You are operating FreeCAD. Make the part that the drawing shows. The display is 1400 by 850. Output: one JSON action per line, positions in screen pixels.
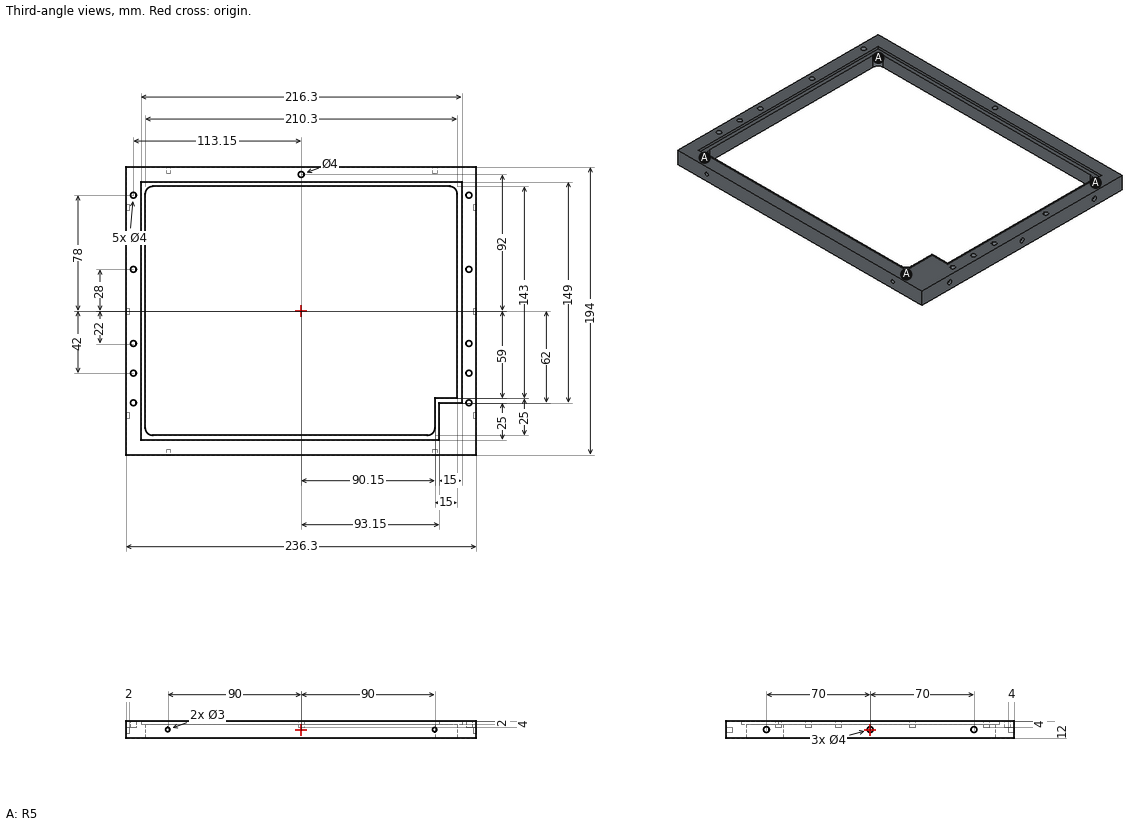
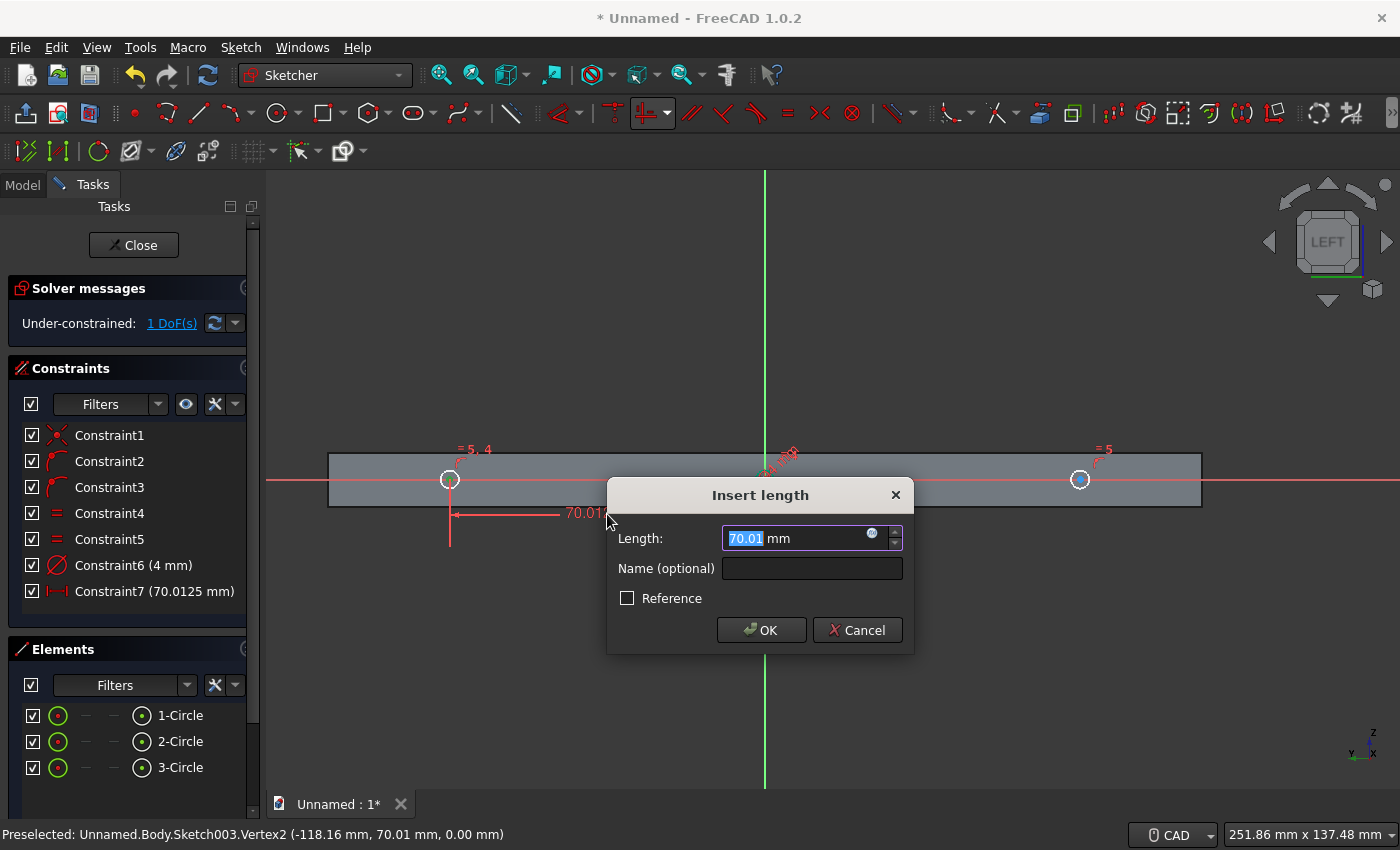
{"action": "type", "text": "70"}
{"action": "key", "text": "Return"}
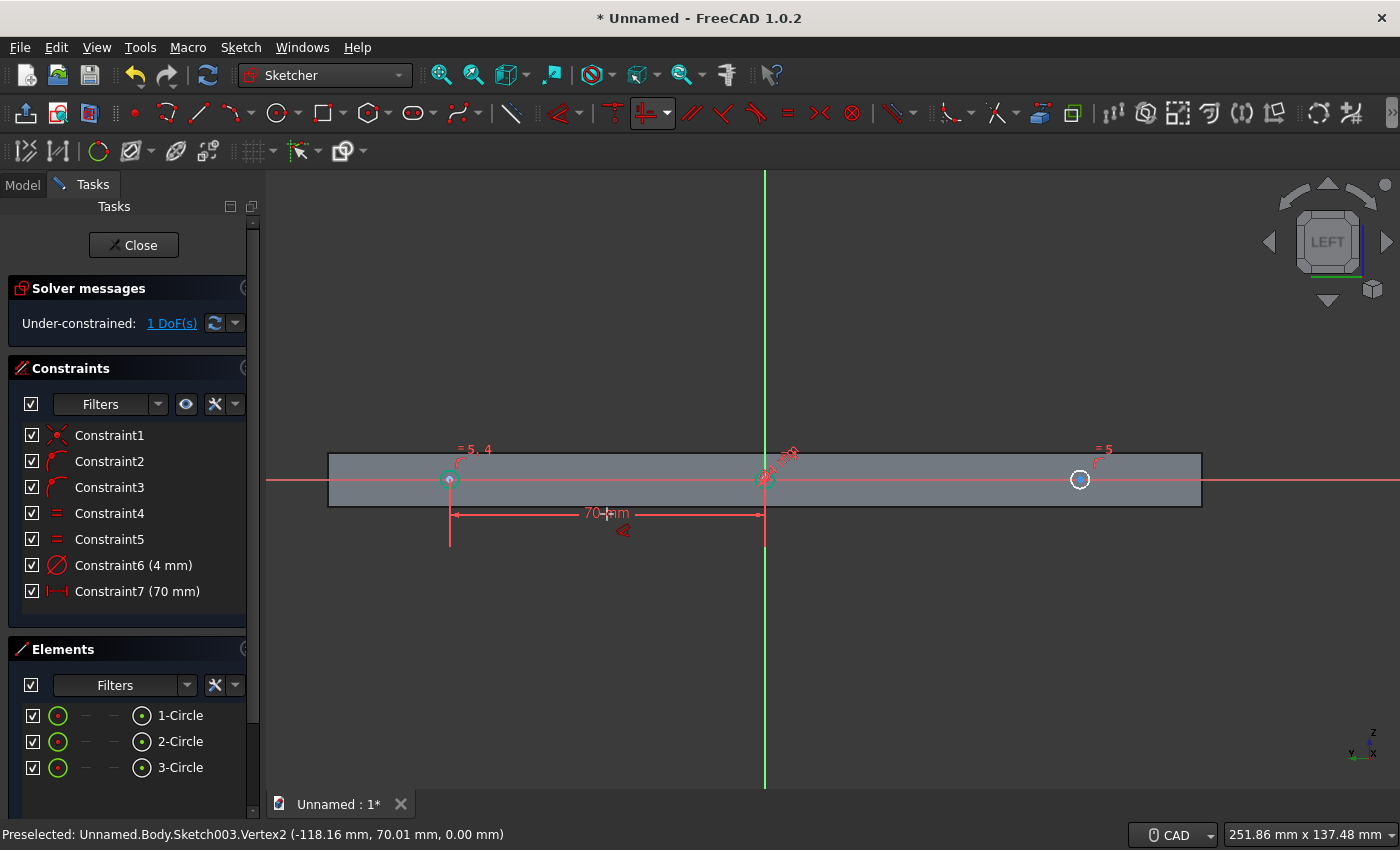
{"action": "left_click", "coordinate": [1080, 480]}
{"action": "left_click", "coordinate": [923, 514]}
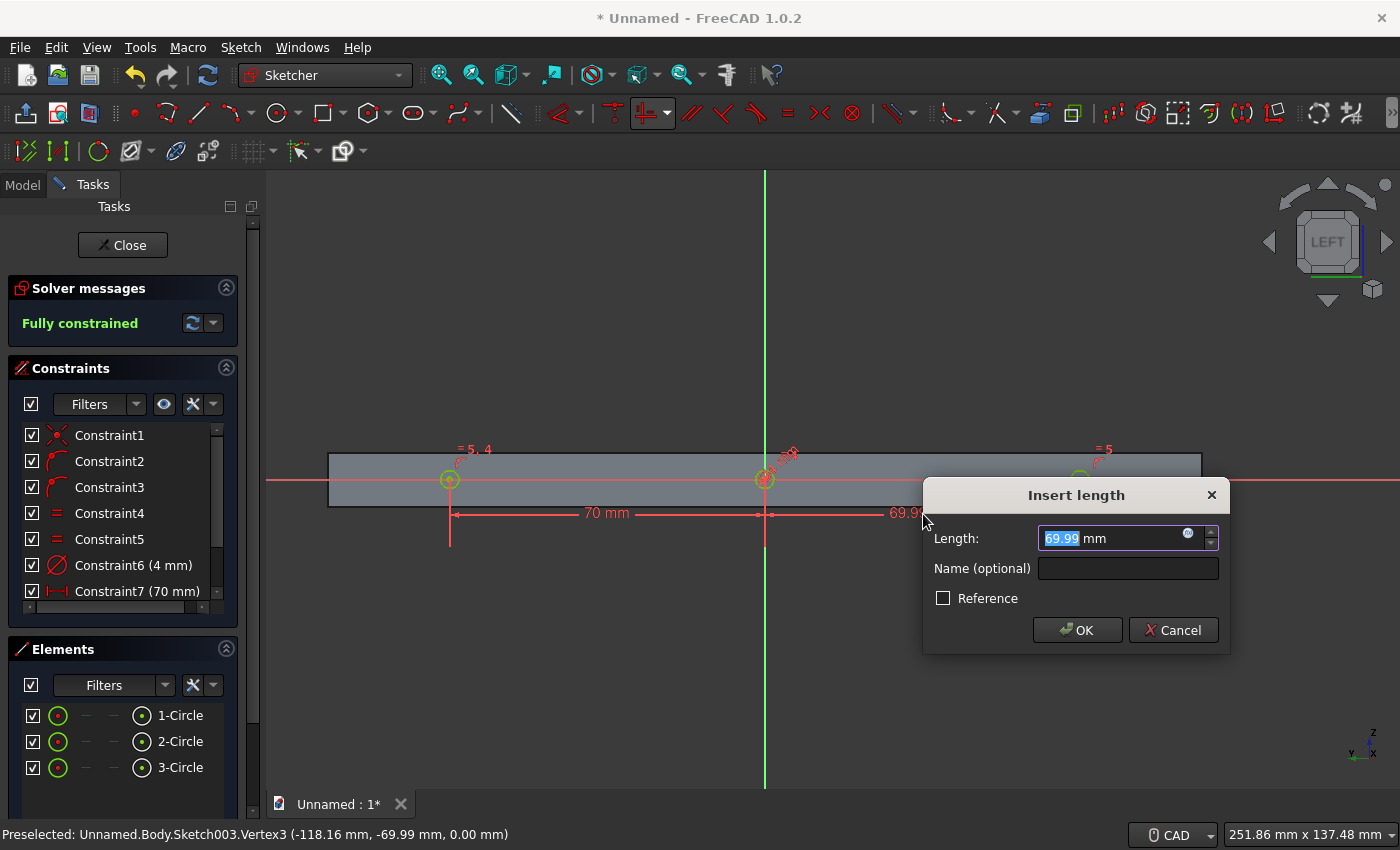
{"action": "type", "text": "70"}
{"action": "key", "text": "Return"}
{"action": "key", "text": "Escape"}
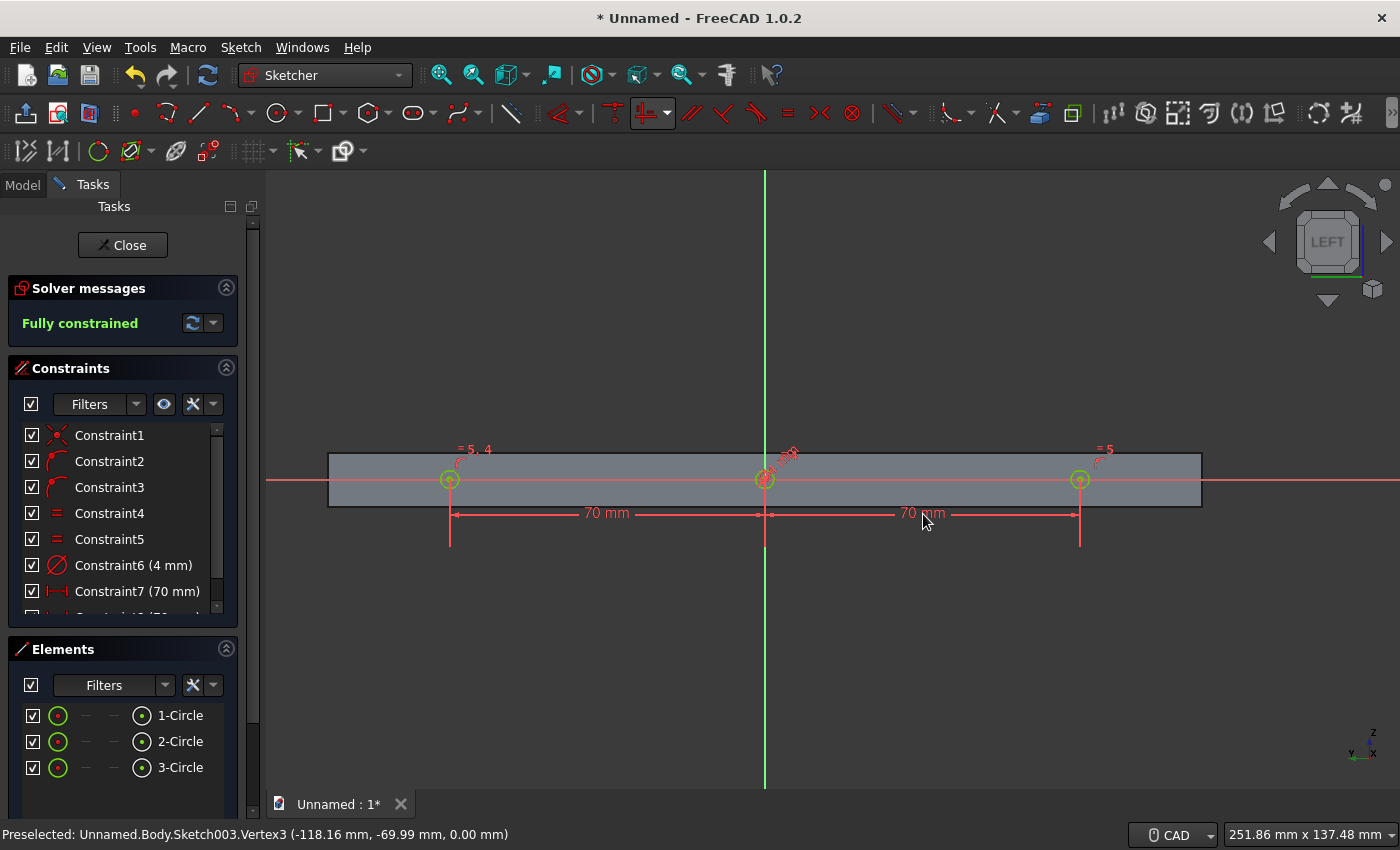
{"action": "left_click", "coordinate": [123, 245]}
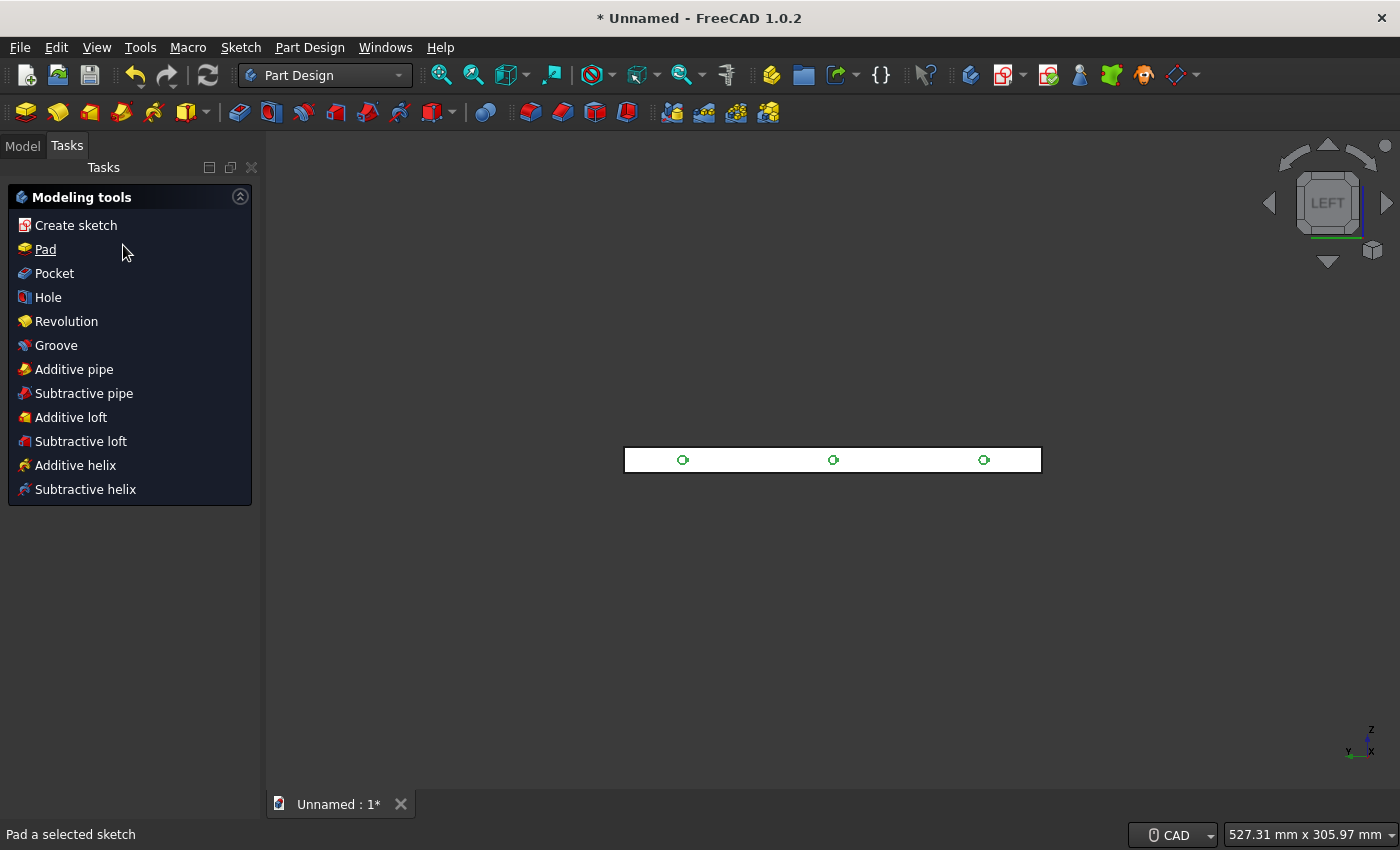
{"action": "left_click", "coordinate": [240, 112]}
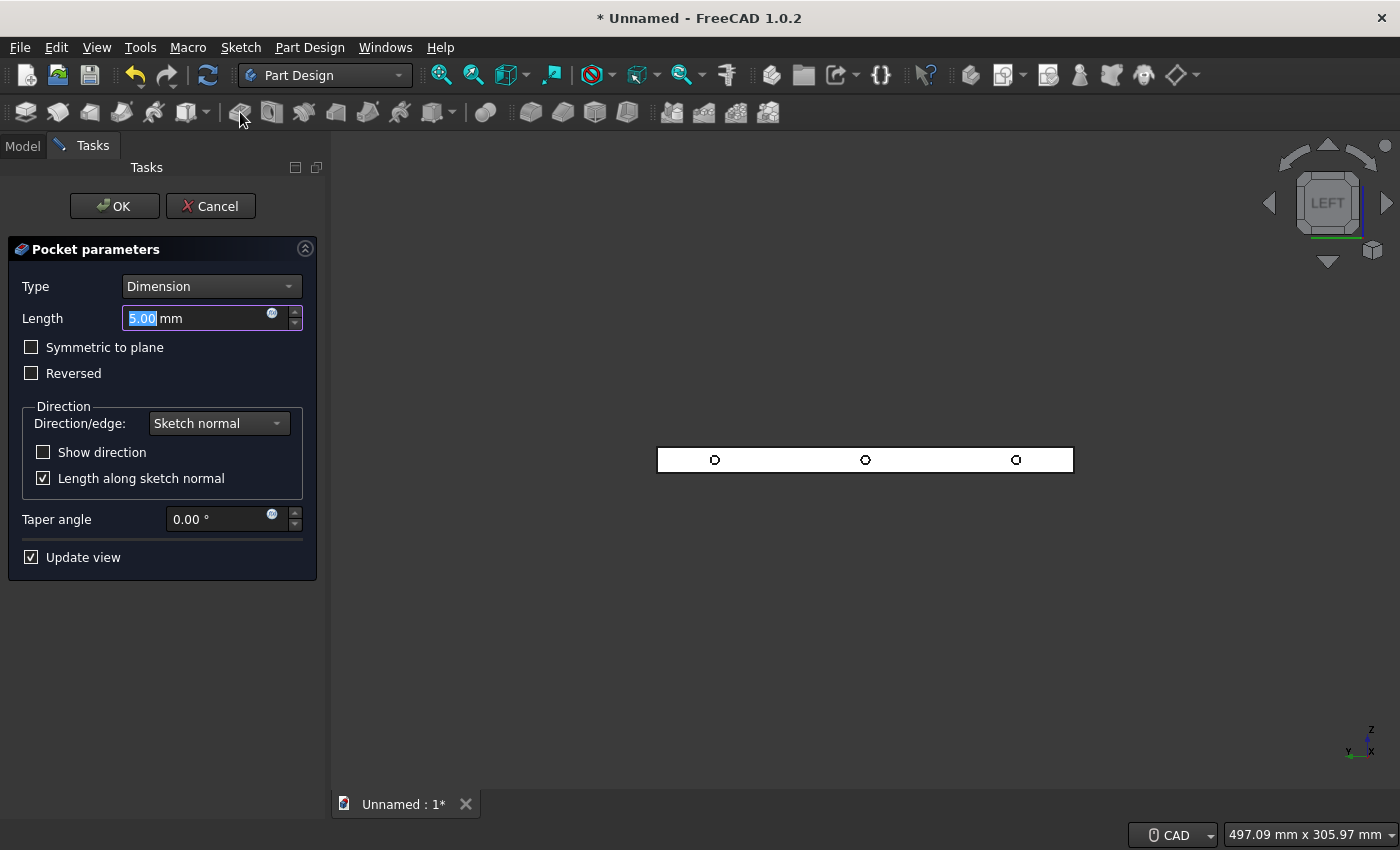
{"action": "type", "text": "2"}
{"action": "key", "text": "Tab"}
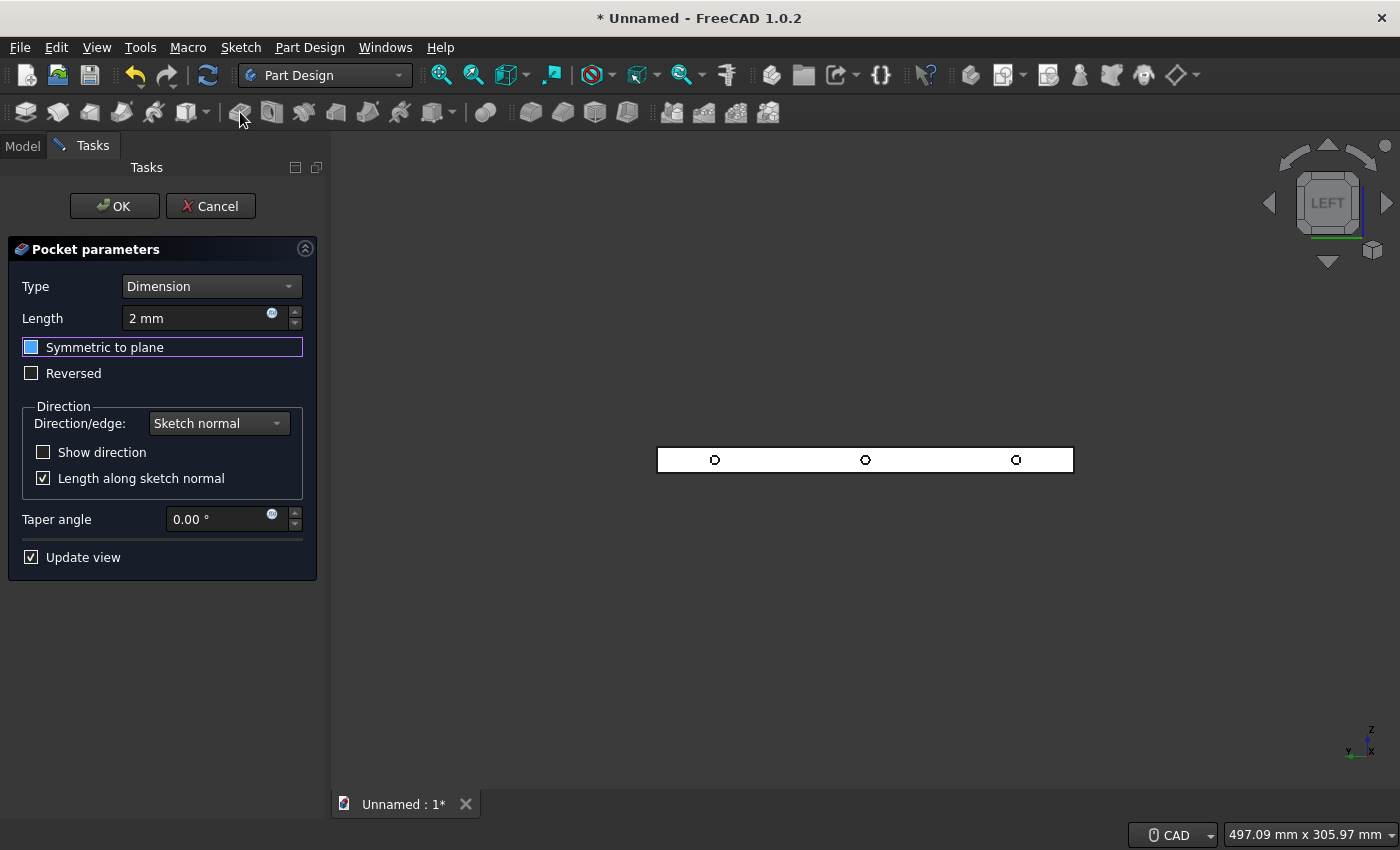
{"action": "left_click", "coordinate": [115, 206]}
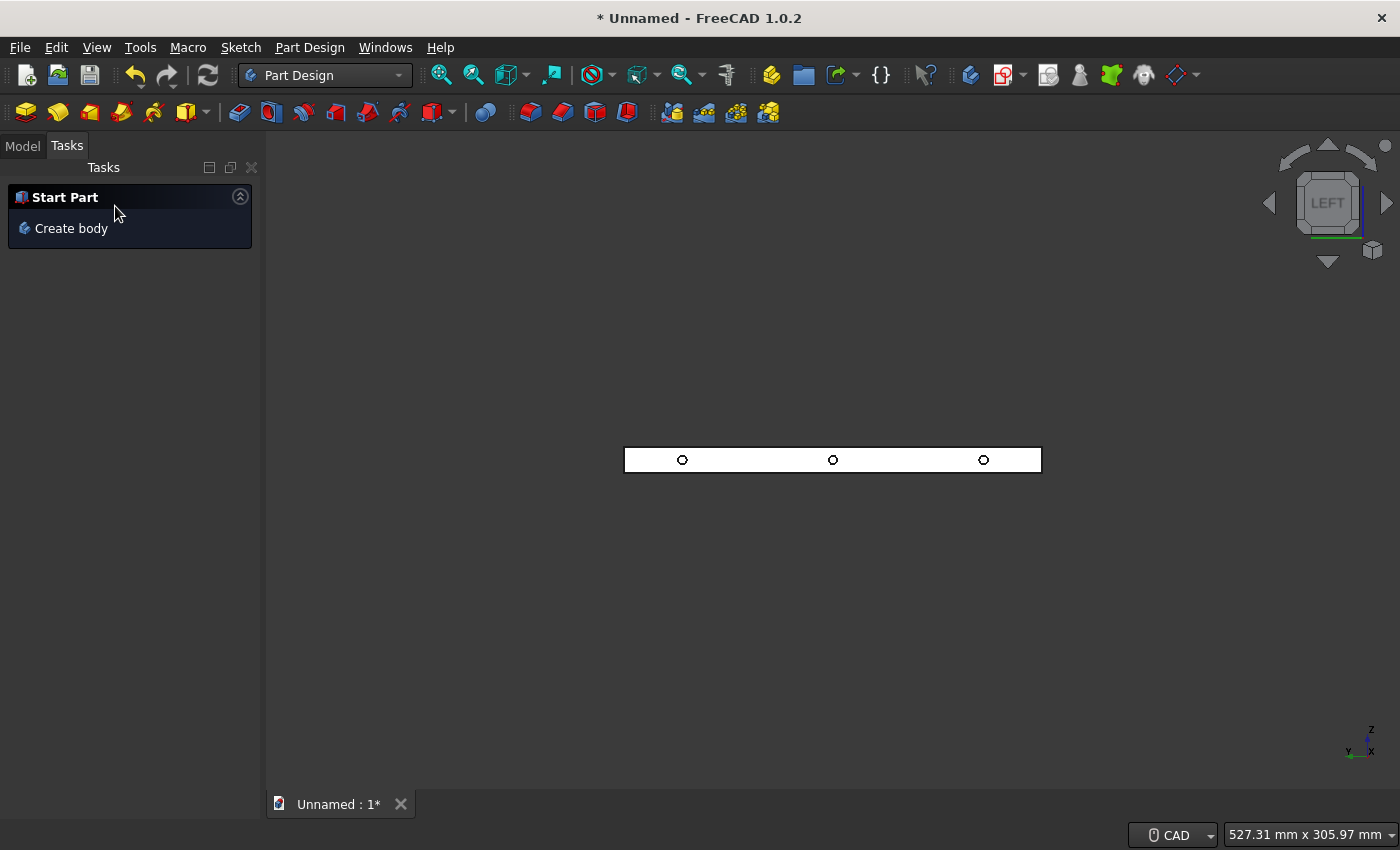
{"action": "left_click", "coordinate": [442, 76]}